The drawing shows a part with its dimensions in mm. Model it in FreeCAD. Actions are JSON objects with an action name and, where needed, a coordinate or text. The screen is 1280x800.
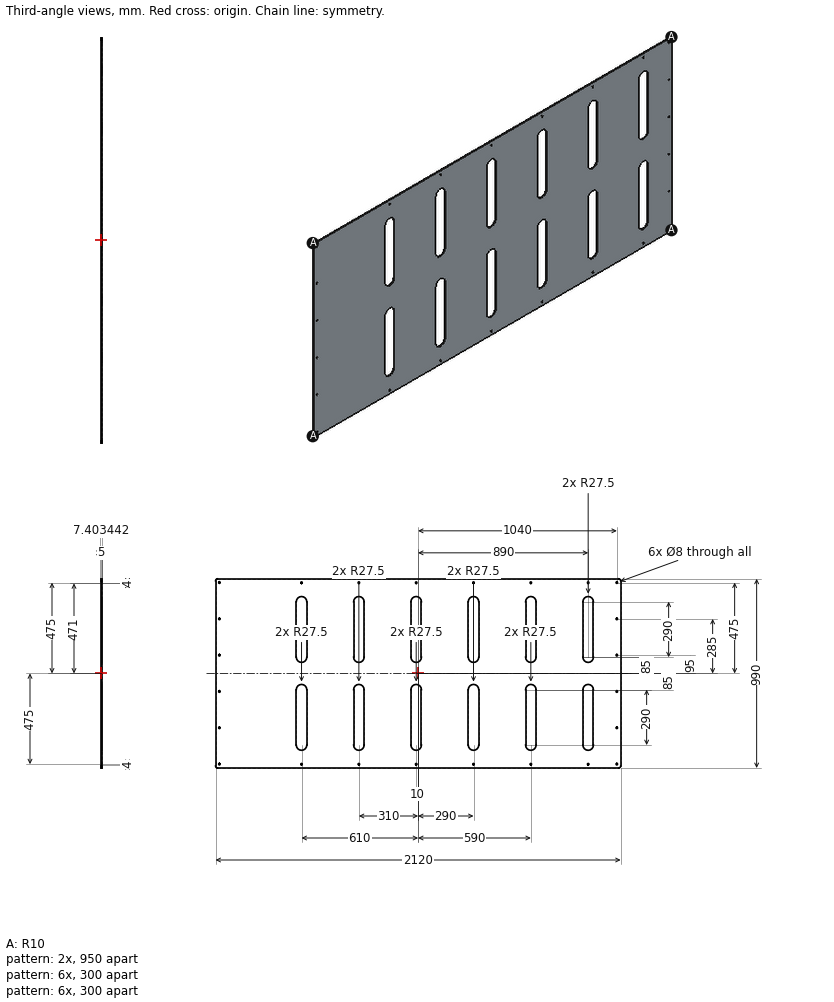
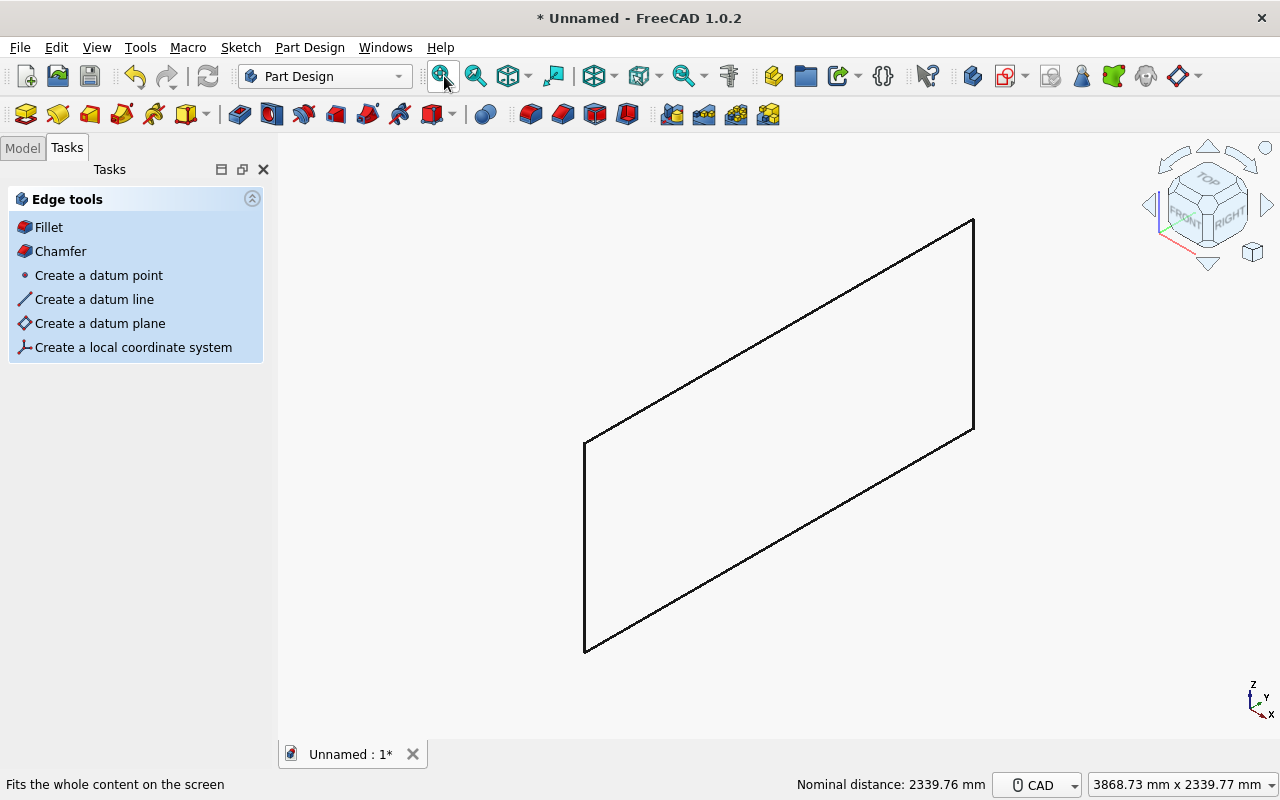
{"action": "scroll", "coordinate": [585, 442], "scroll_direction": "up", "scroll_amount": 15}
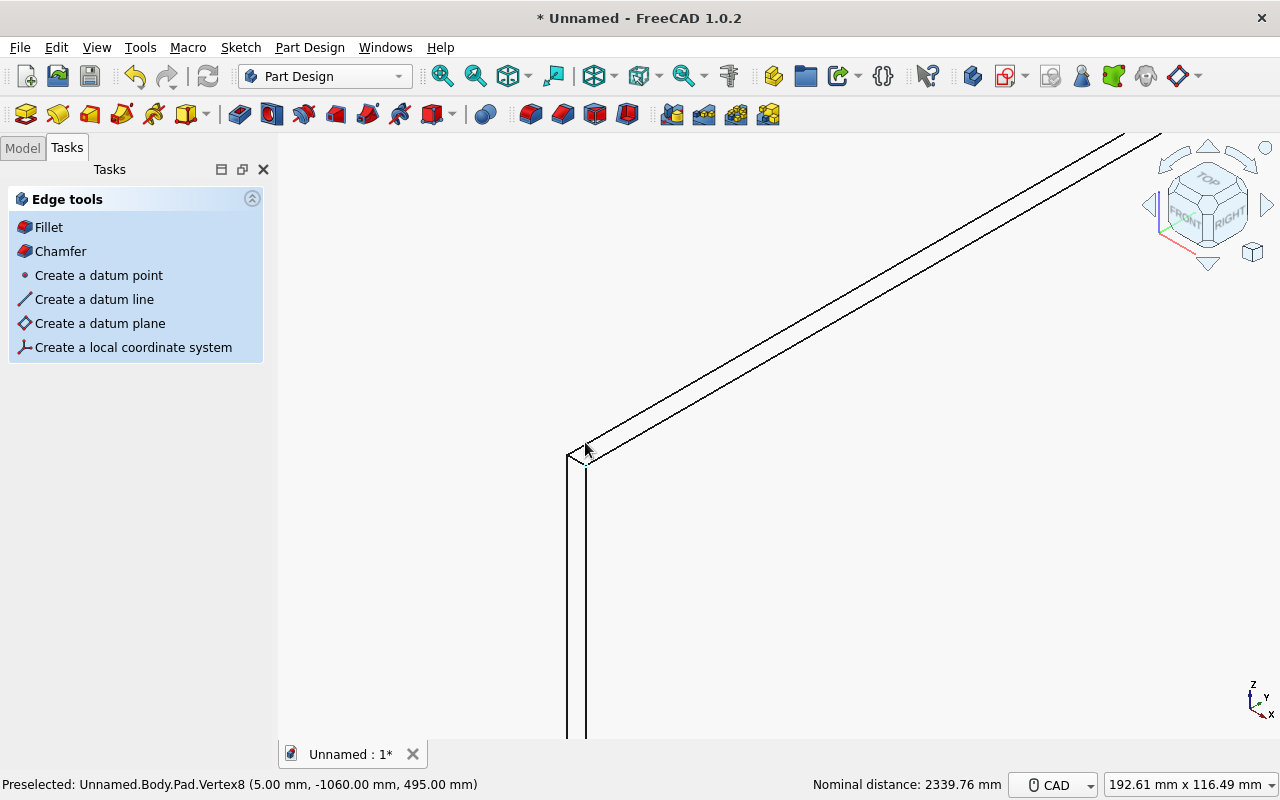
{"action": "left_click", "coordinate": [577, 459], "text": "ctrl"}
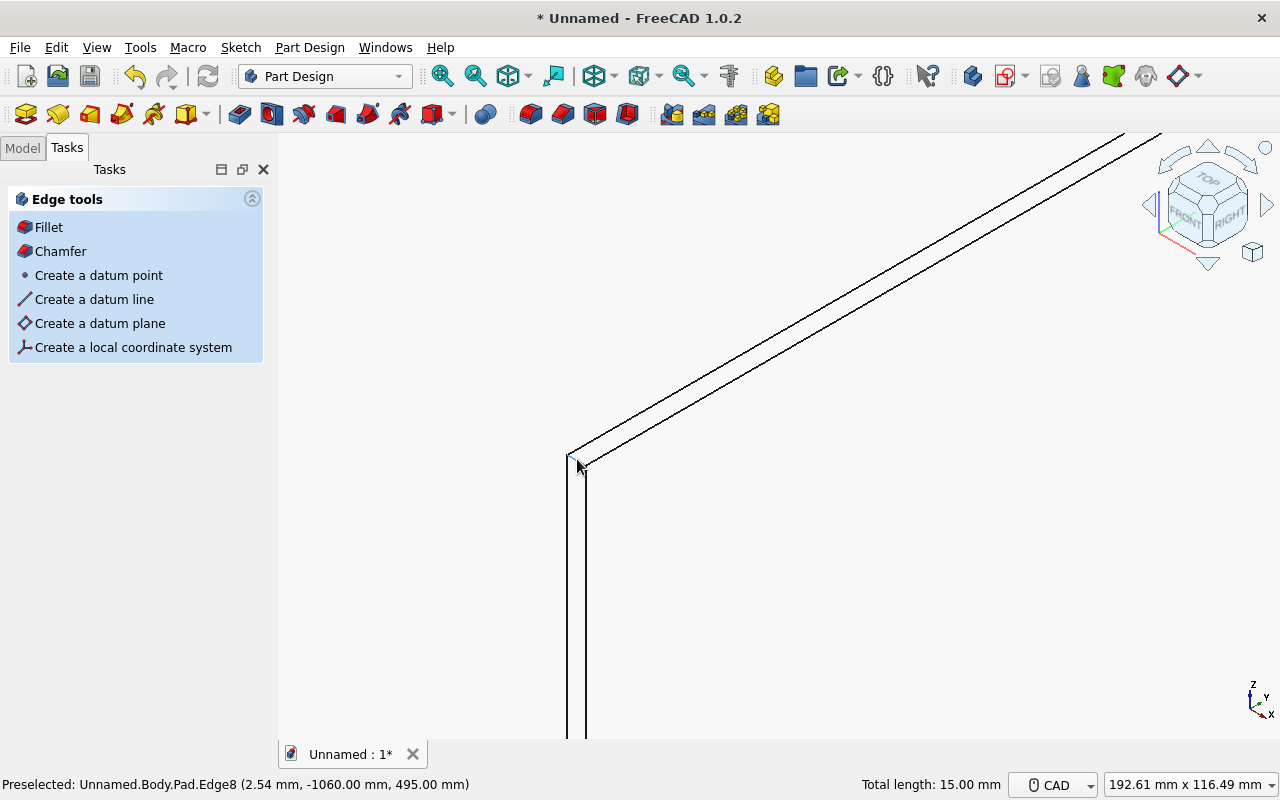
{"action": "key", "text": "v f"}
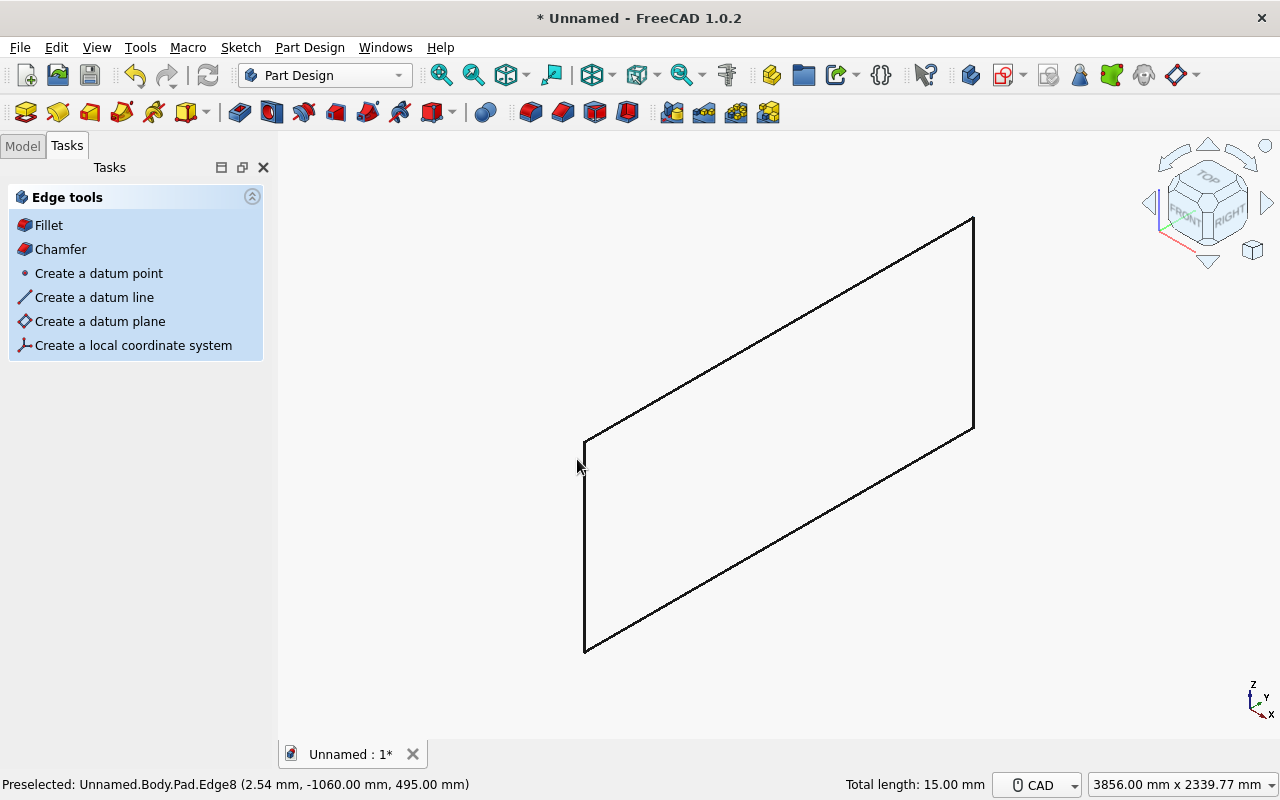
{"action": "key", "text": "2"}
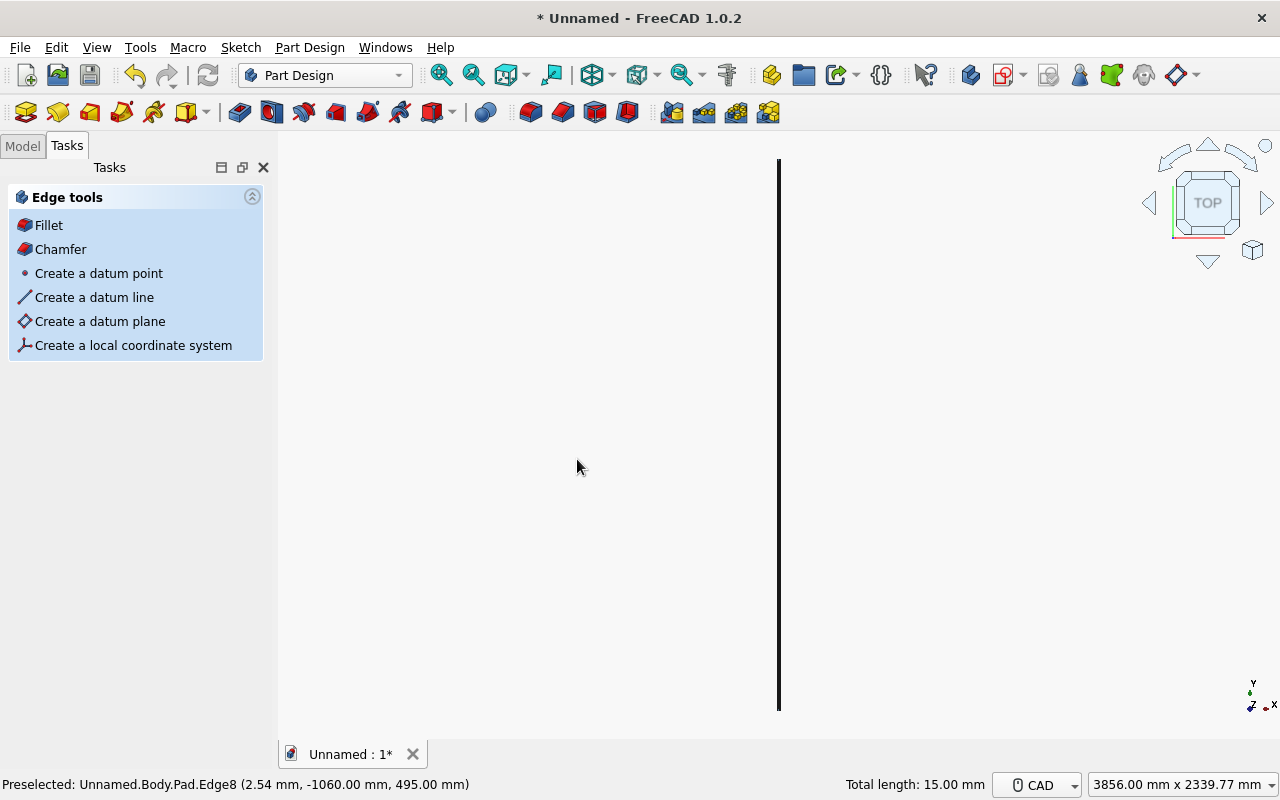
{"action": "key", "text": "1"}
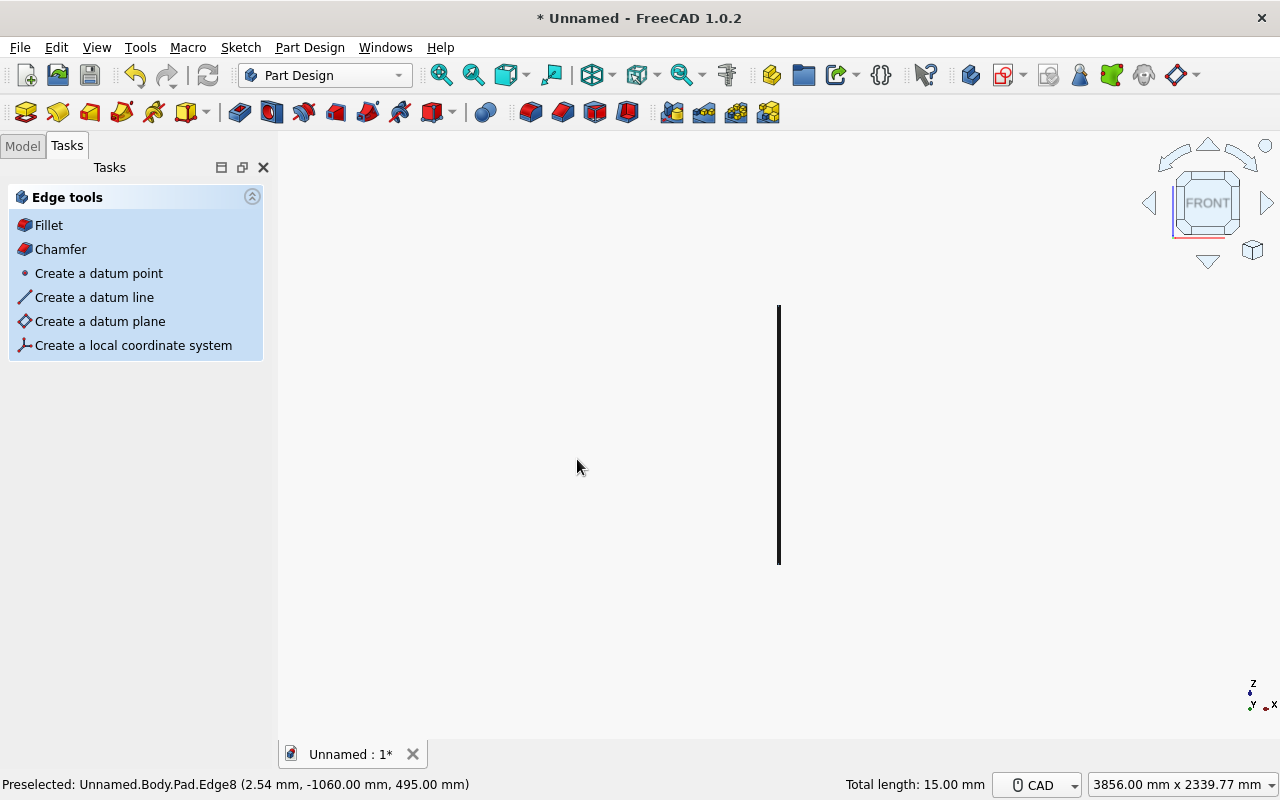
{"action": "left_click", "coordinate": [442, 76]}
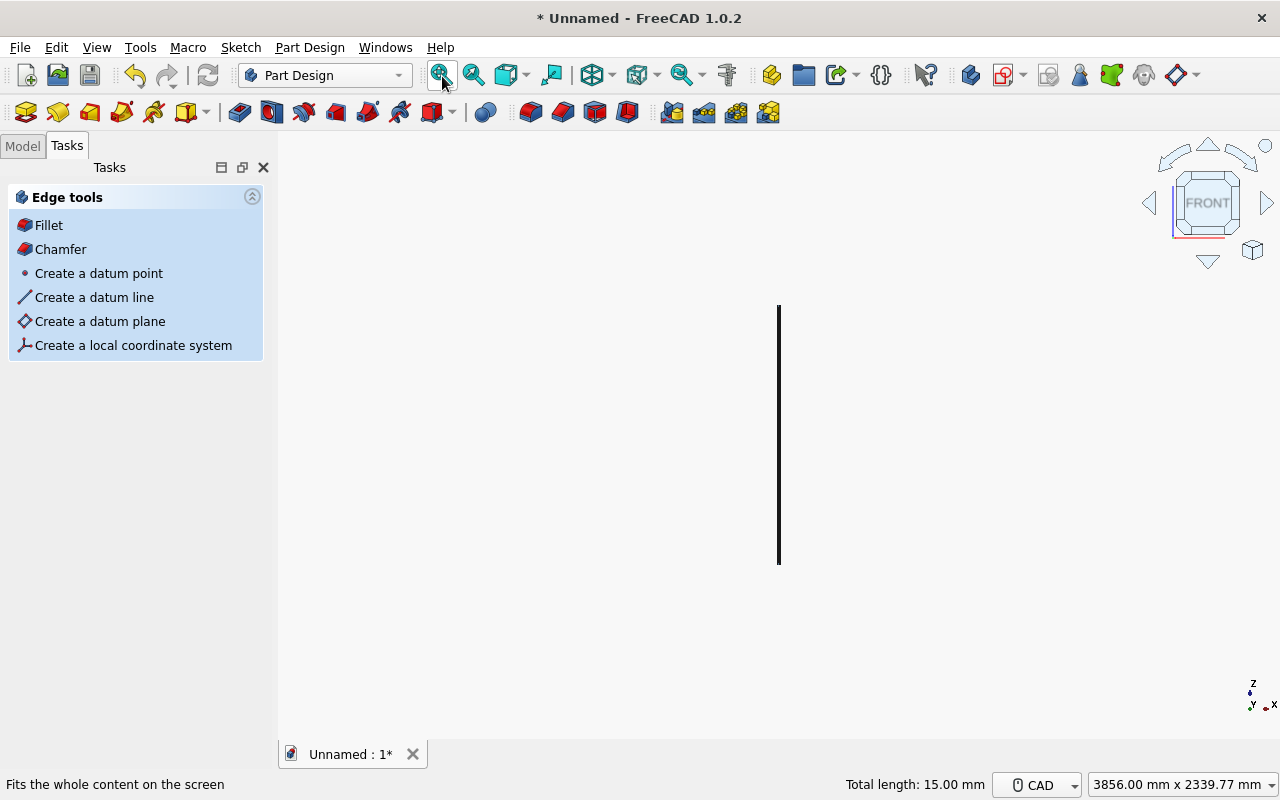
{"action": "scroll", "coordinate": [779, 563], "scroll_direction": "up", "scroll_amount": 15}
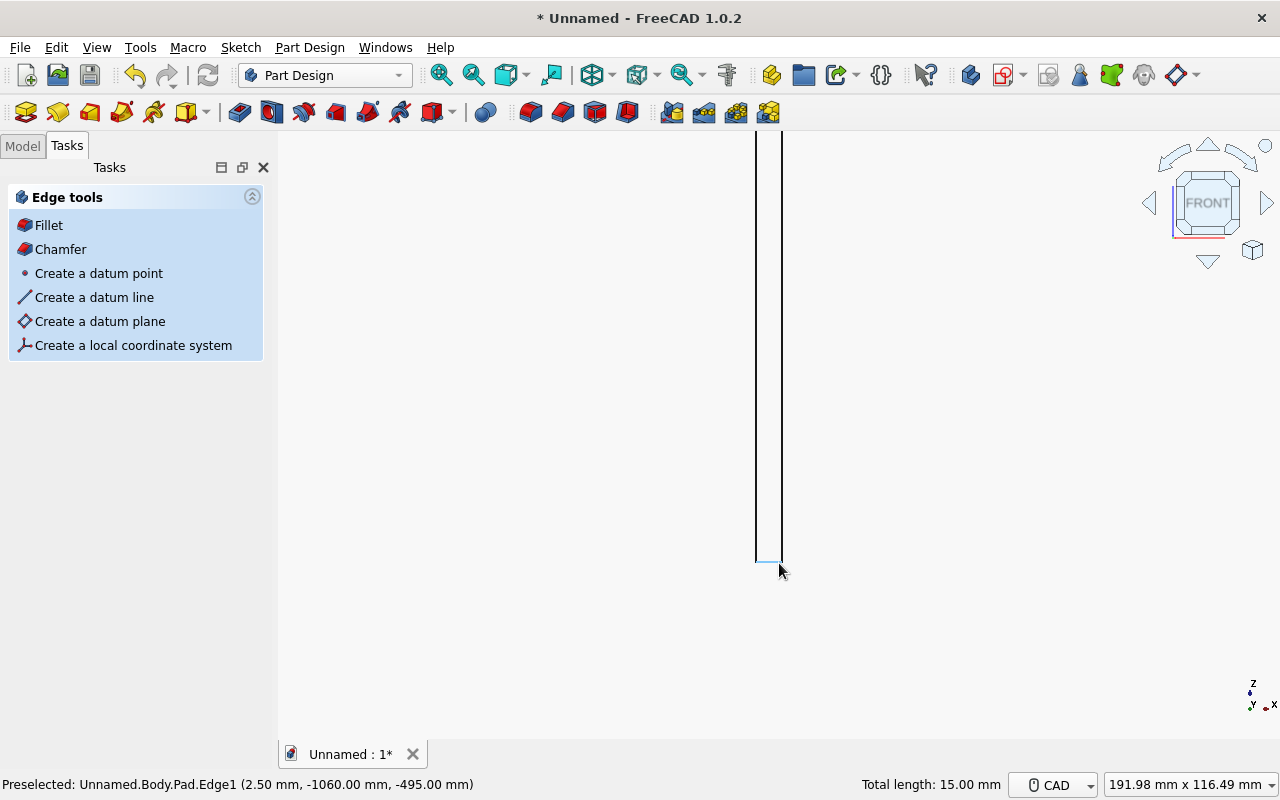
{"action": "left_click", "coordinate": [442, 76]}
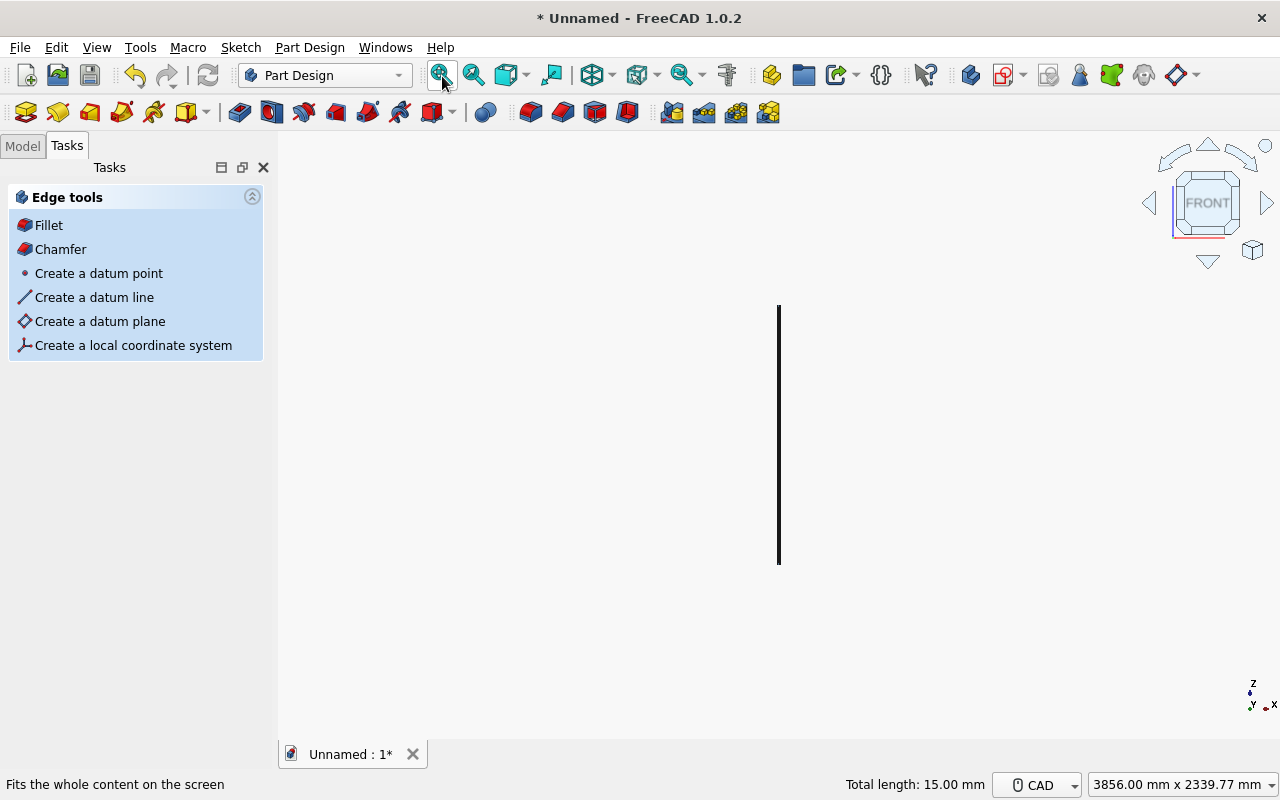
{"action": "key", "text": "3"}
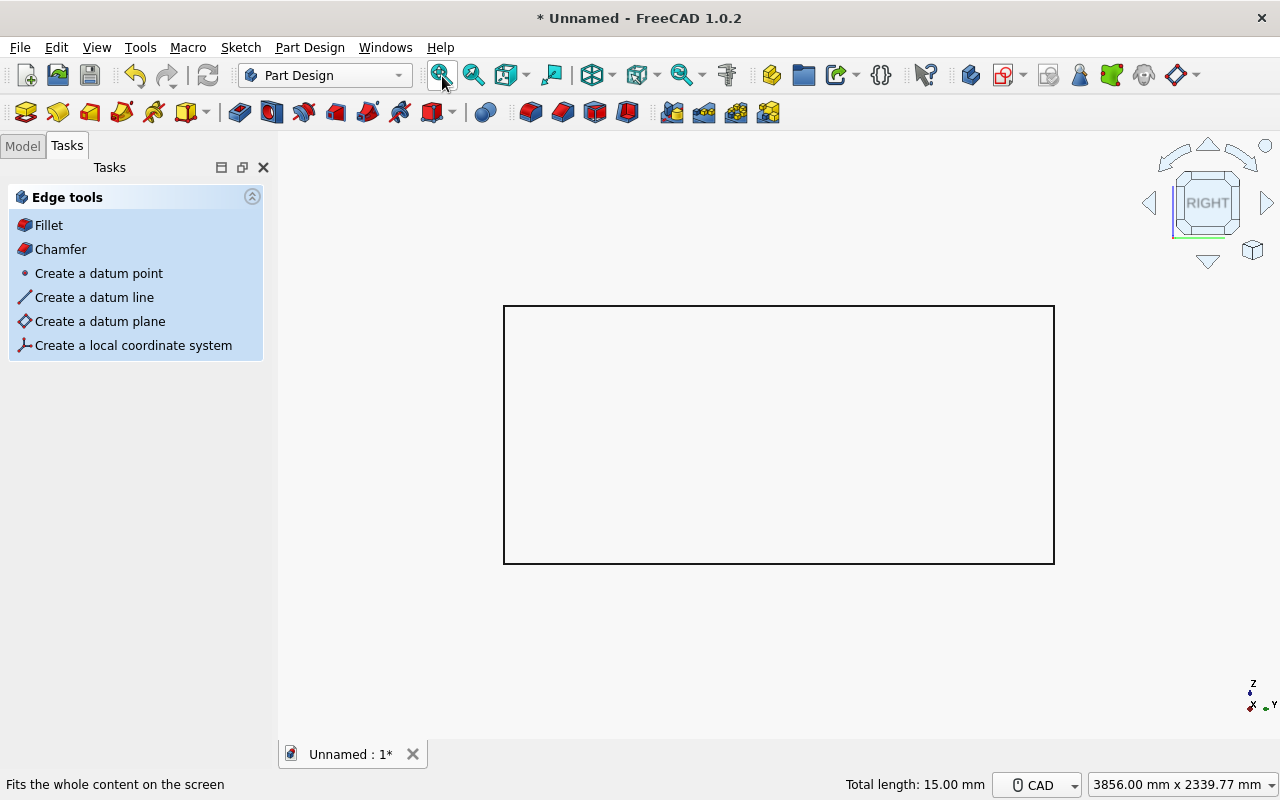
{"action": "scroll", "coordinate": [1054, 563], "scroll_direction": "up", "scroll_amount": 15}